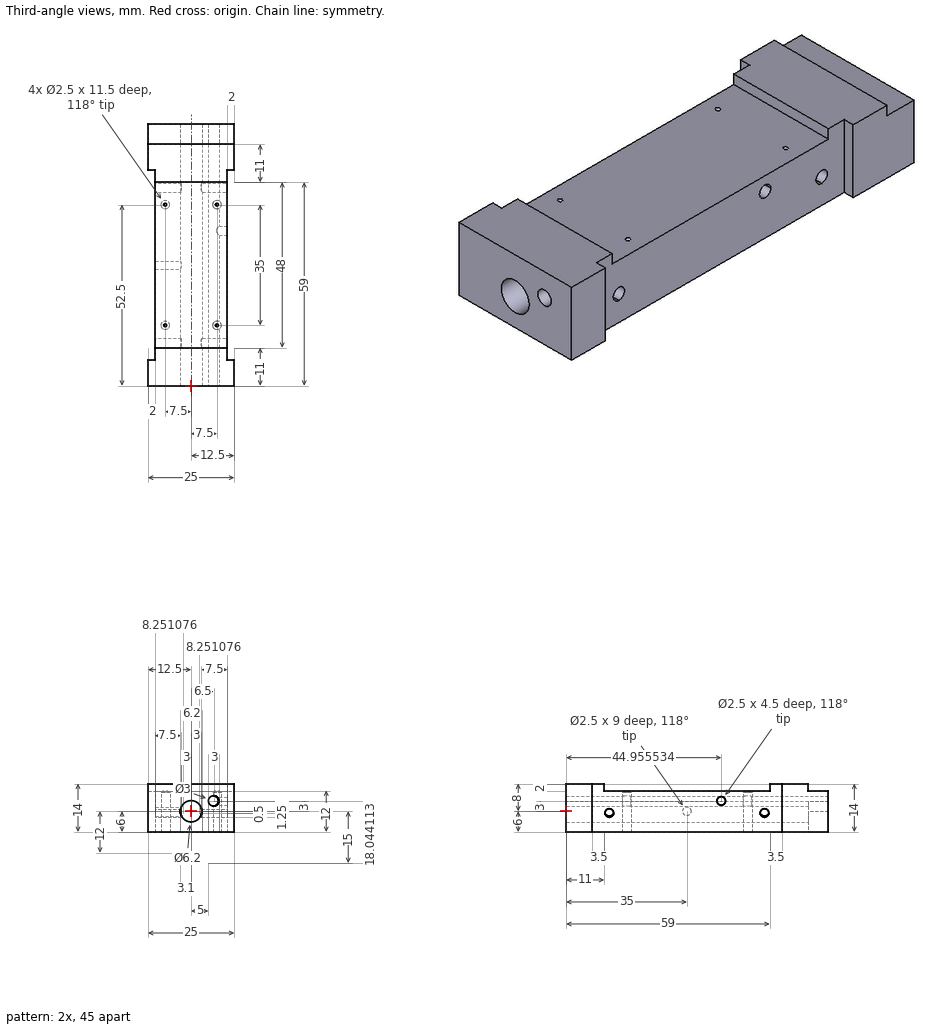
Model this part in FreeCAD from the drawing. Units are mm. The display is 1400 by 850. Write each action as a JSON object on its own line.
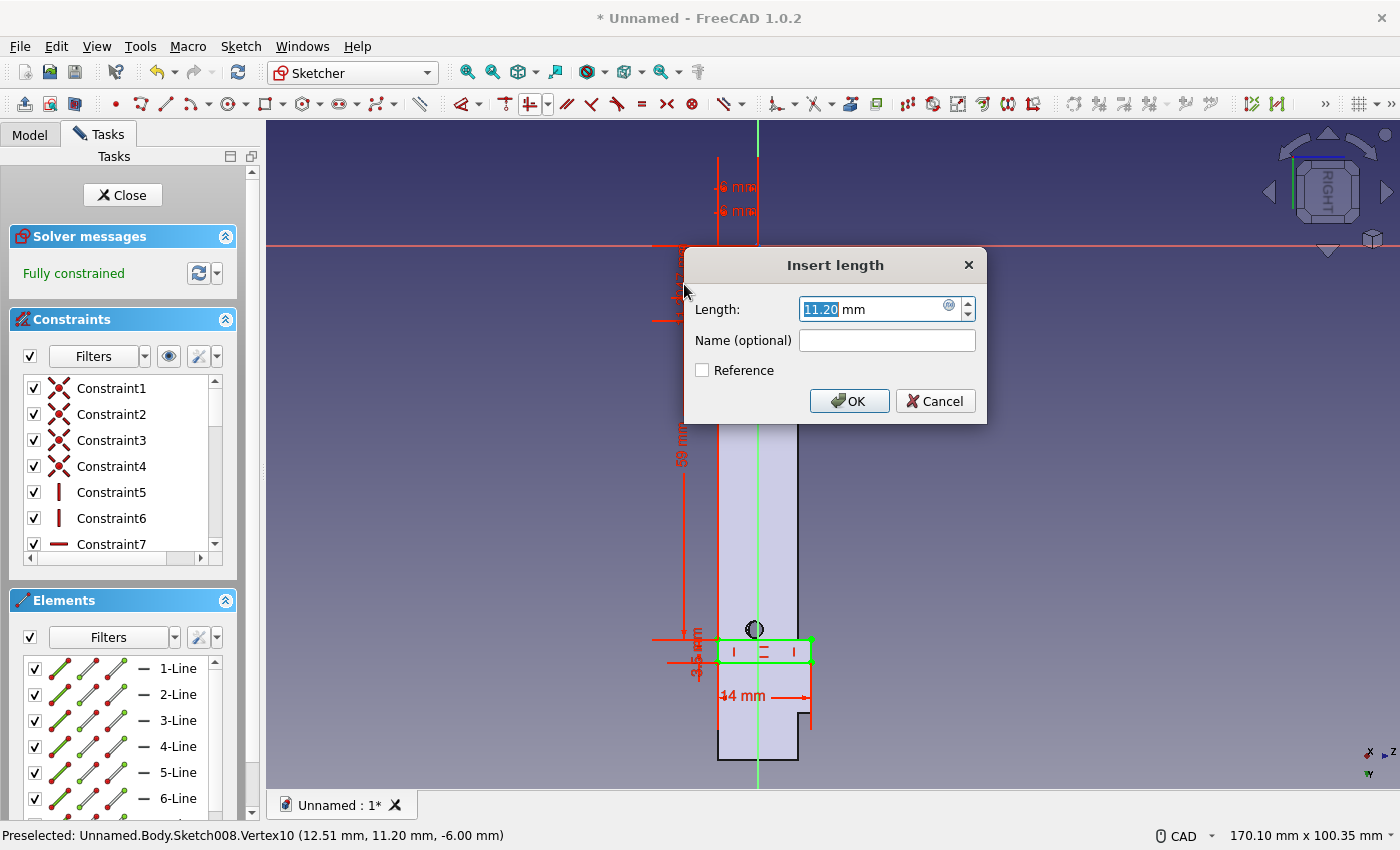
{"action": "type", "text": "11"}
{"action": "key", "text": "Return"}
{"action": "key", "text": "Escape"}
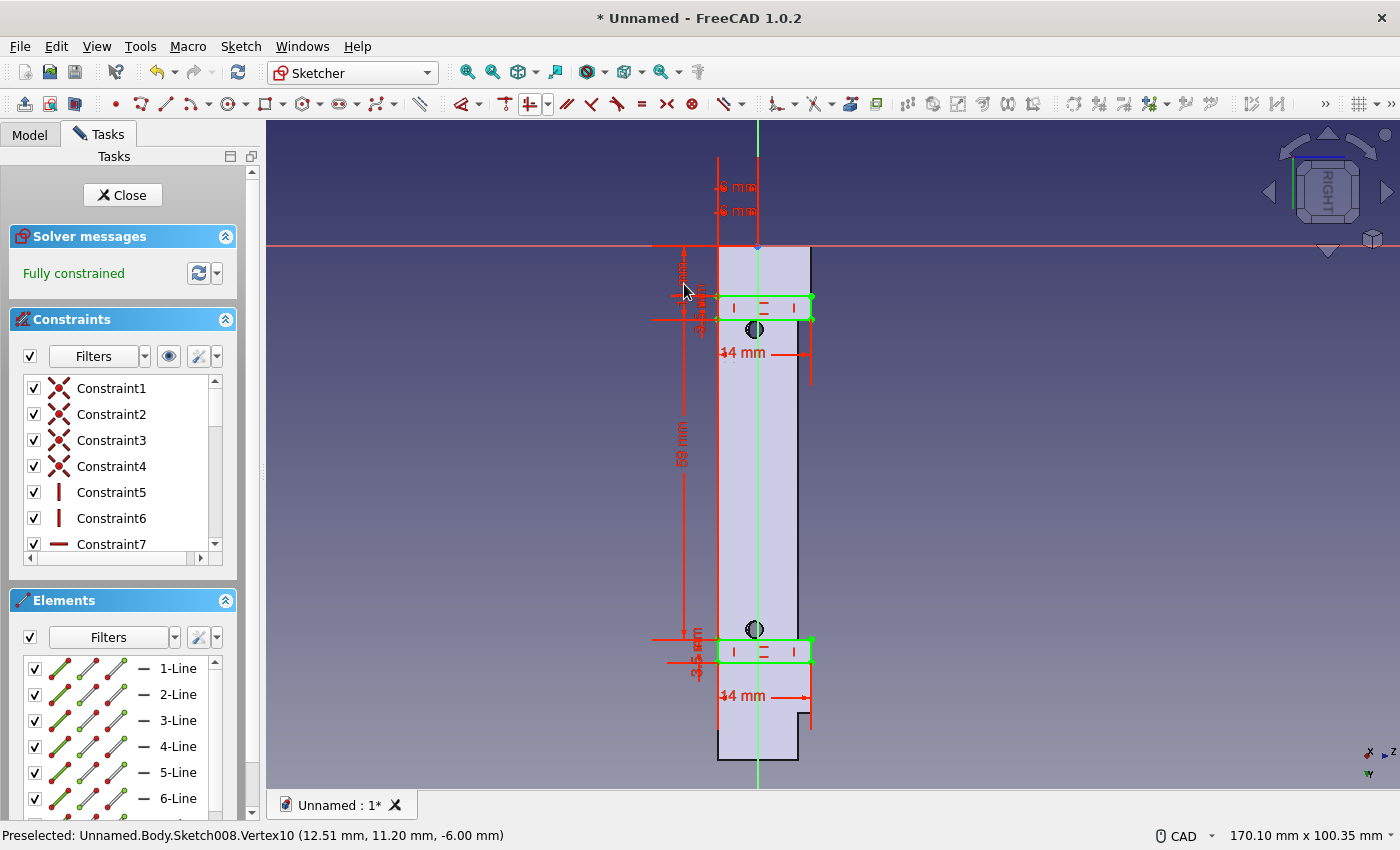
{"action": "left_click", "coordinate": [123, 195]}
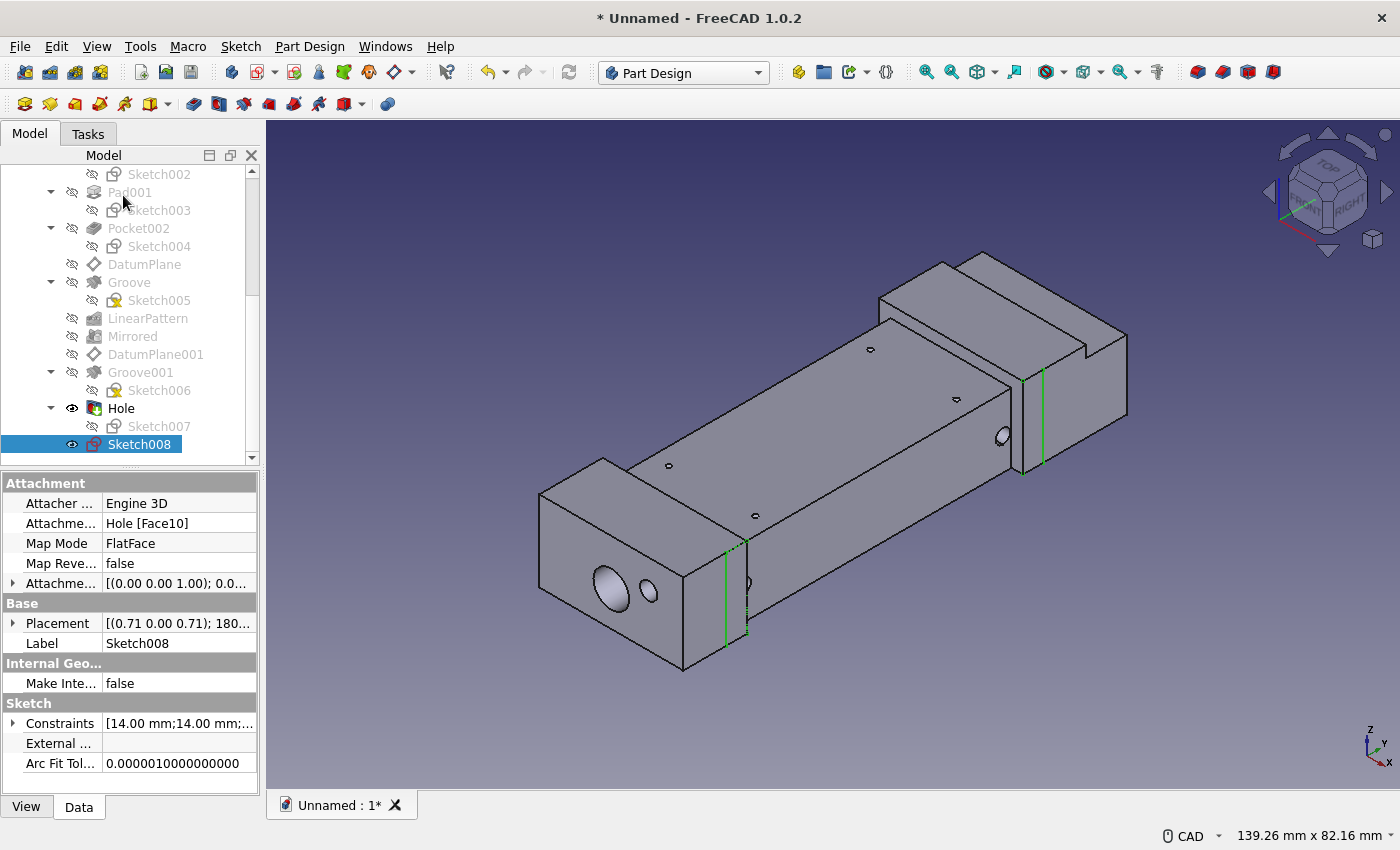
{"action": "left_click", "coordinate": [194, 104]}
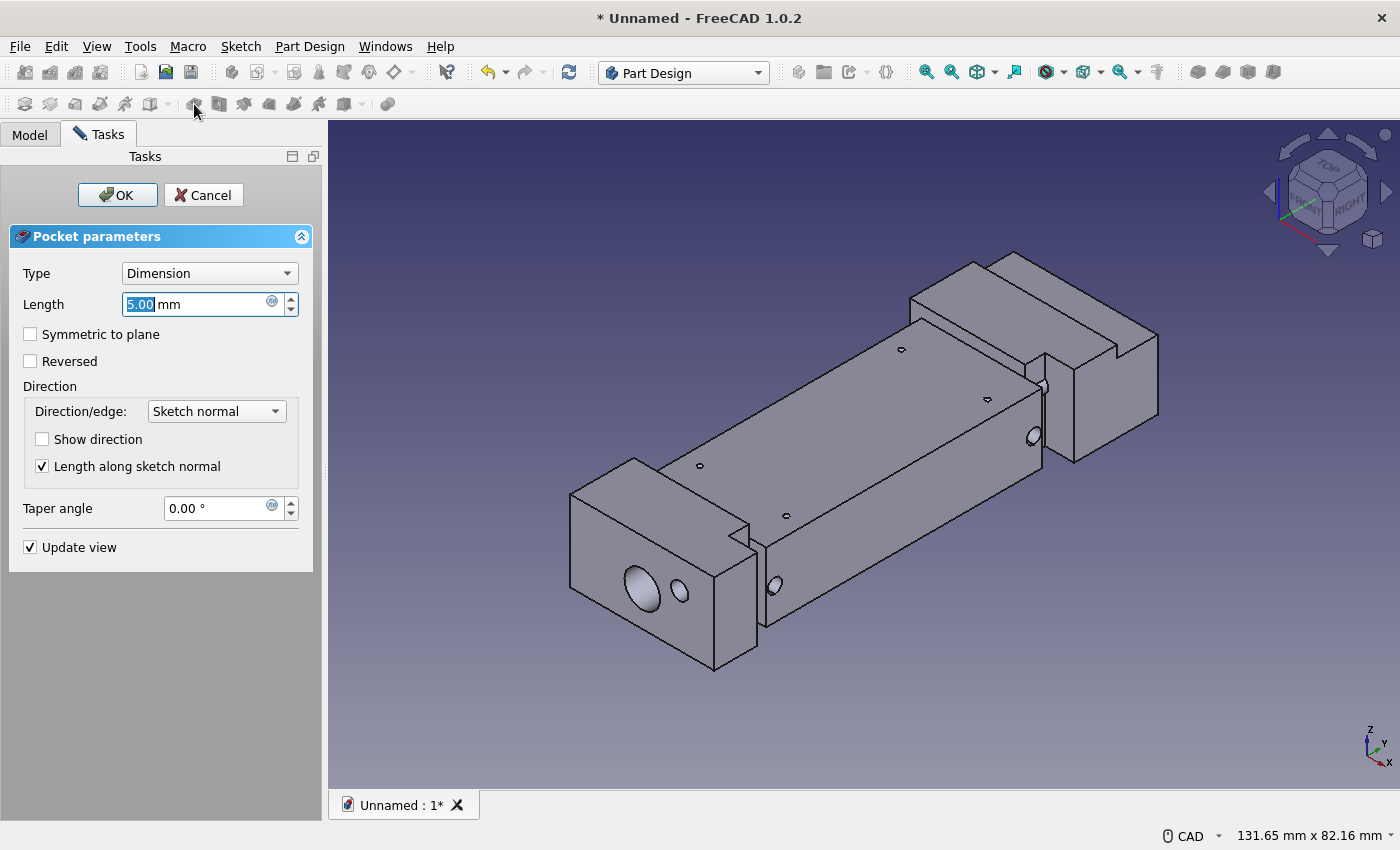
{"action": "type", "text": "2"}
{"action": "key", "text": "Tab"}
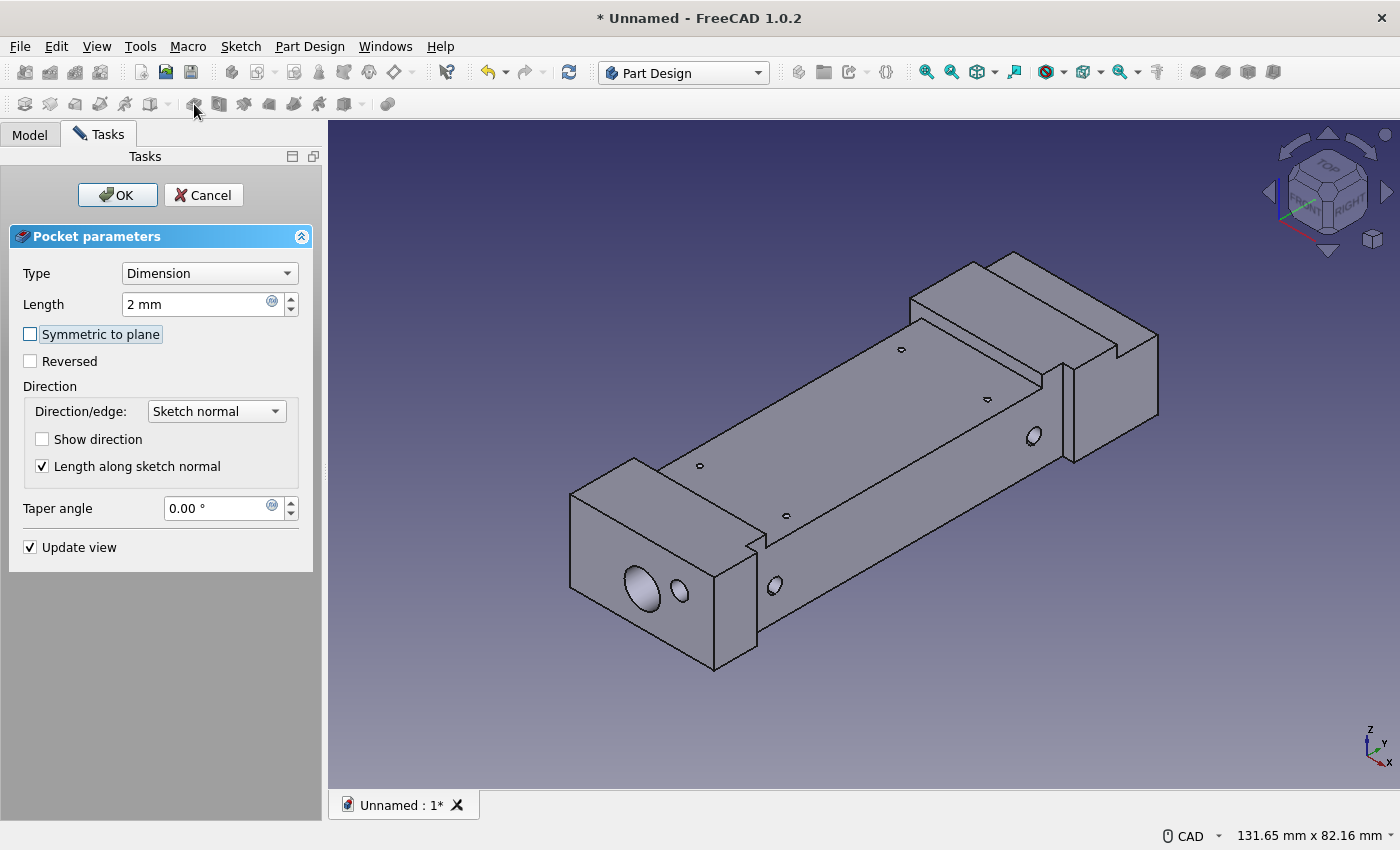
{"action": "left_click", "coordinate": [118, 195]}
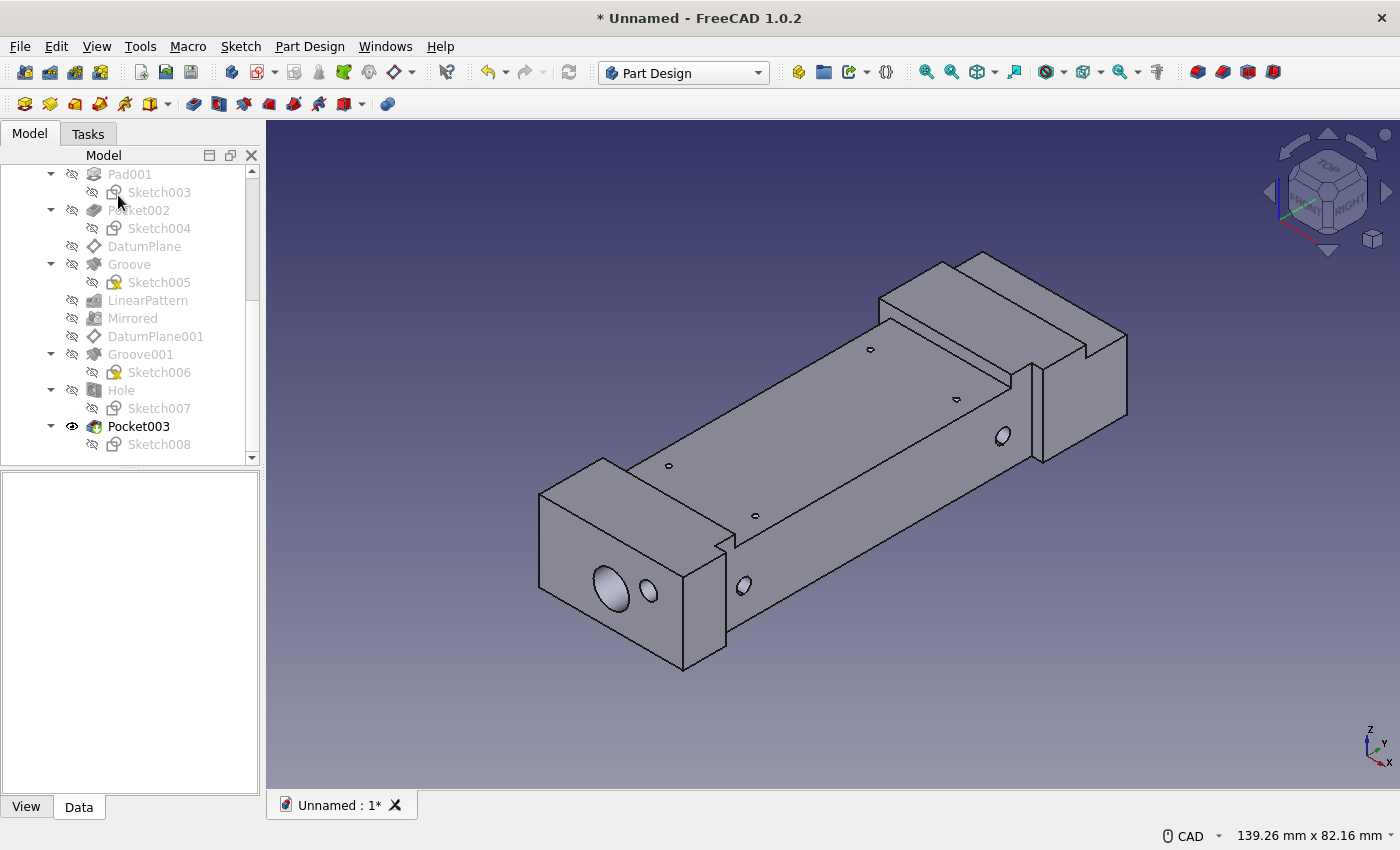
{"action": "key", "text": "6"}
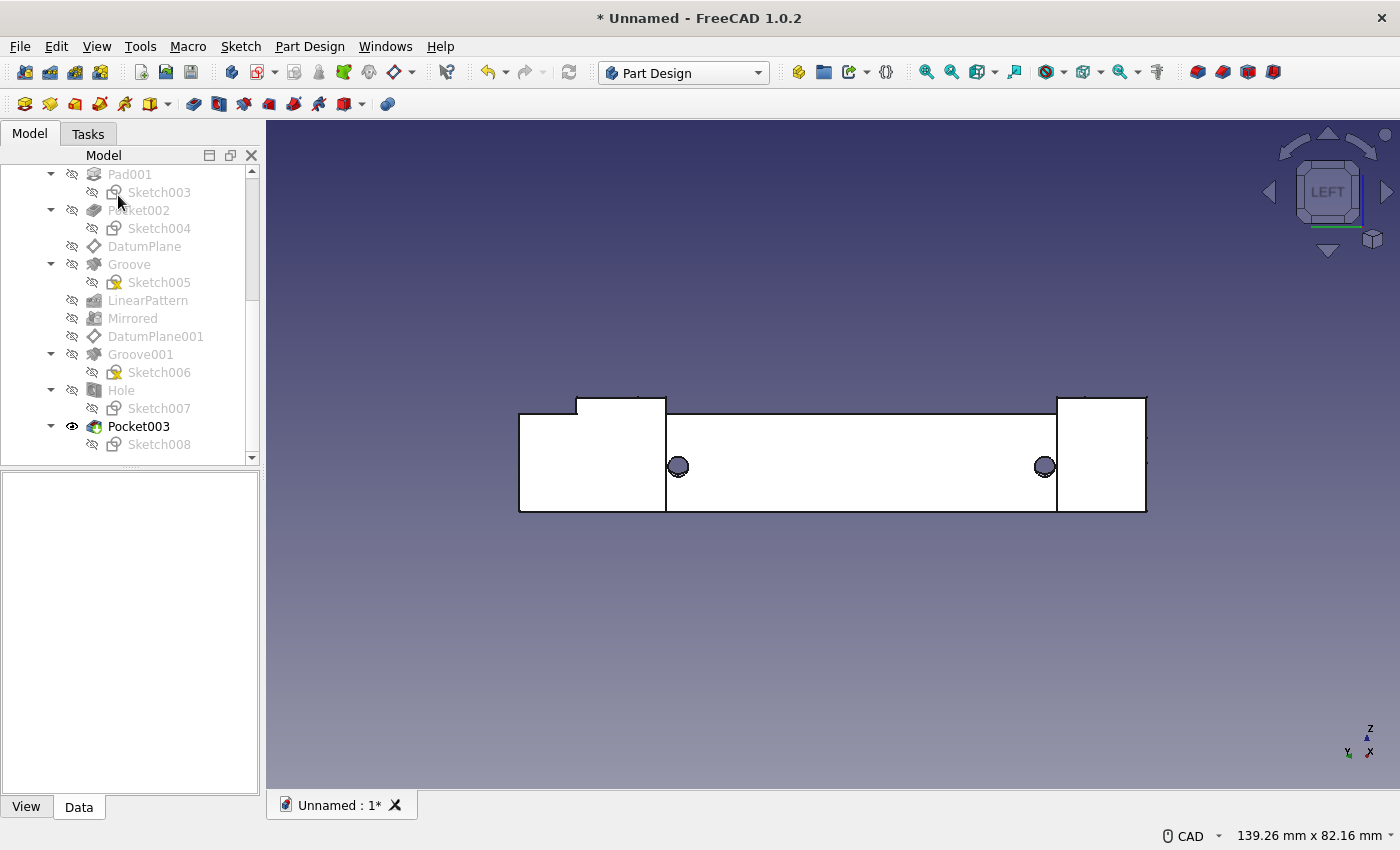
{"action": "left_click", "coordinate": [614, 454]}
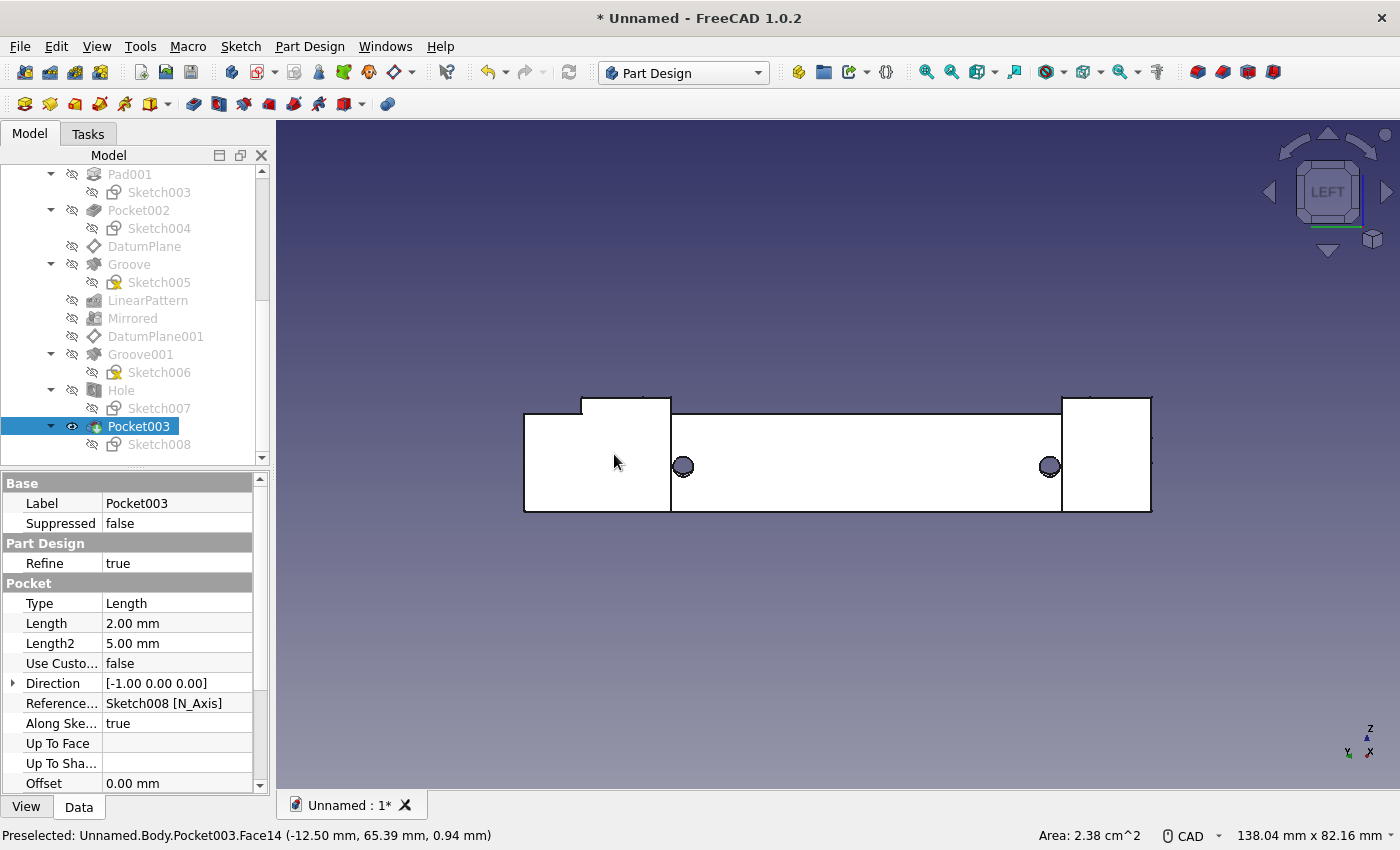
{"action": "left_click", "coordinate": [256, 72]}